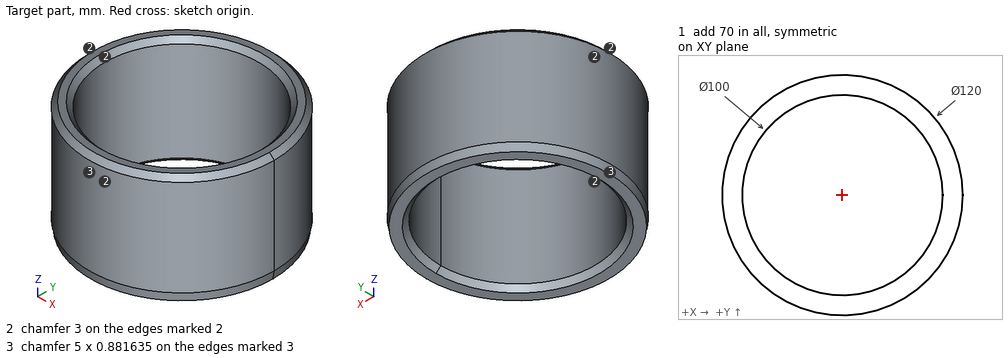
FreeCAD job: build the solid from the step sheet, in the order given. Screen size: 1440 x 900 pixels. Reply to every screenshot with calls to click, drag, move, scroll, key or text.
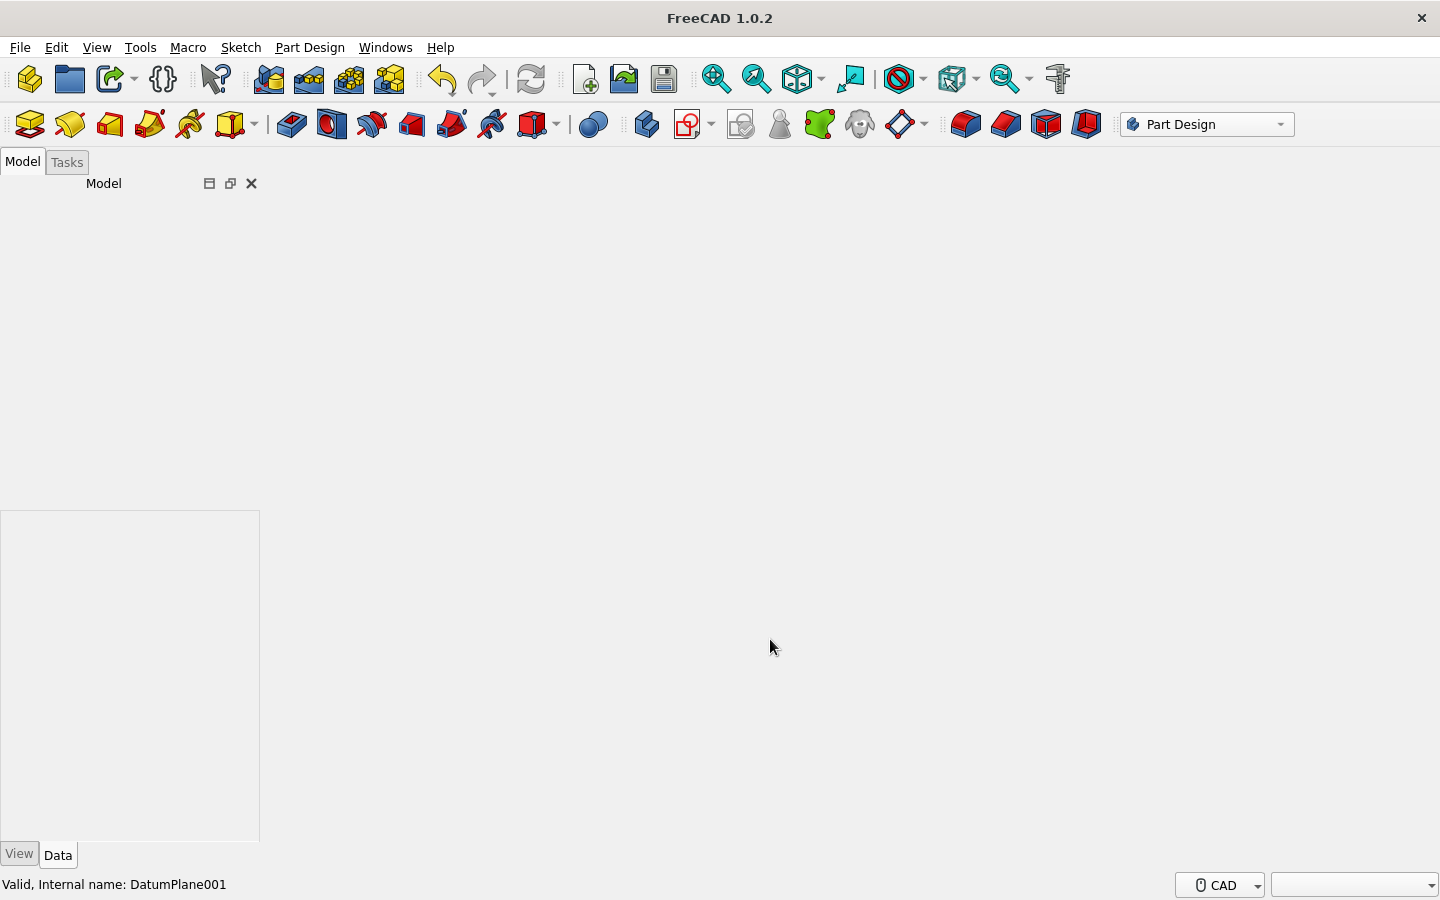
click(584, 80)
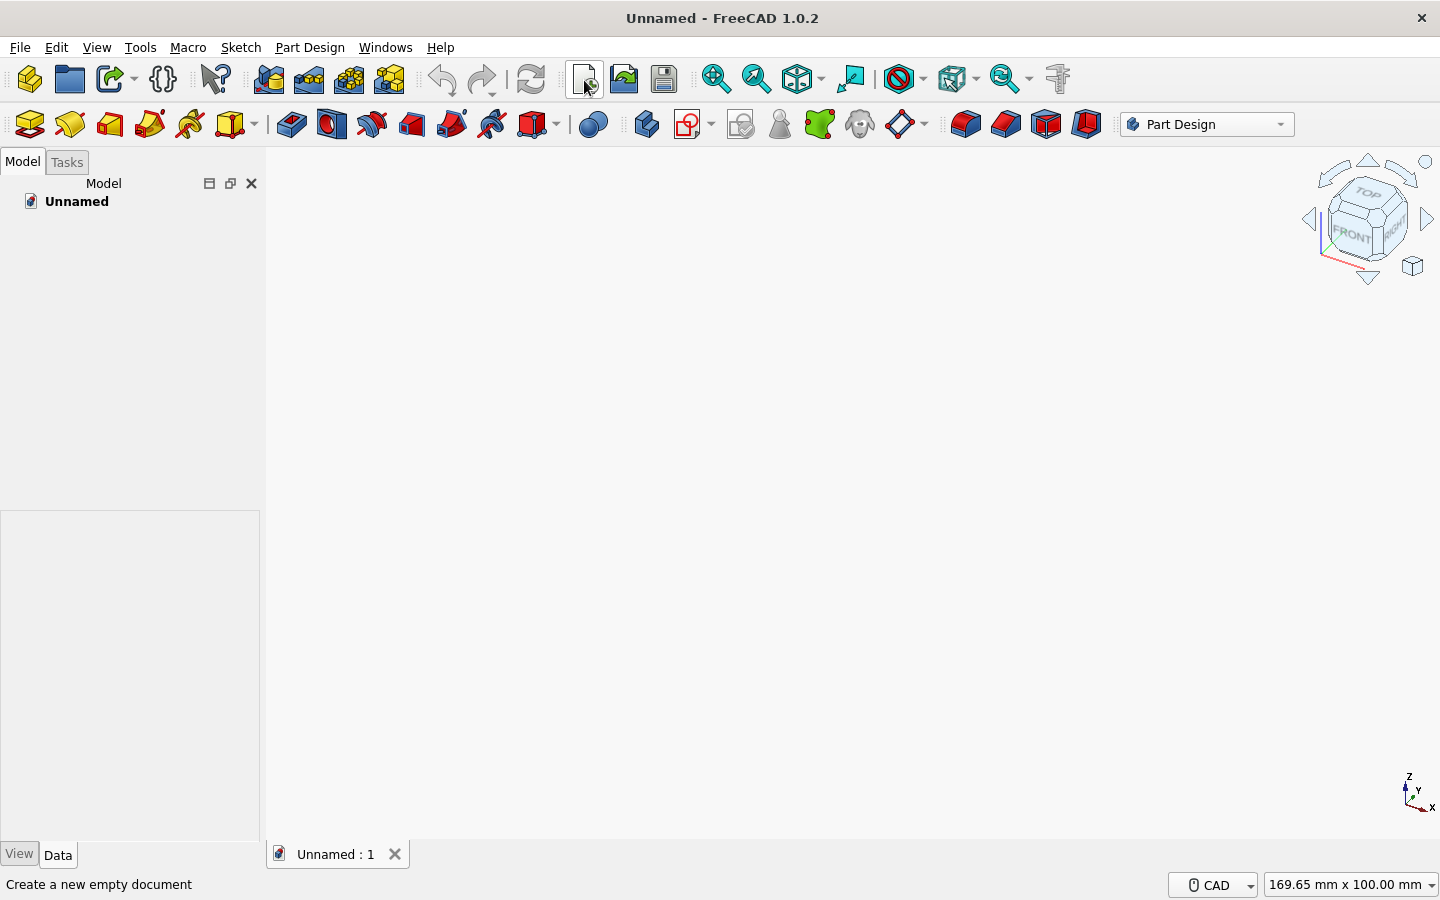
click(688, 124)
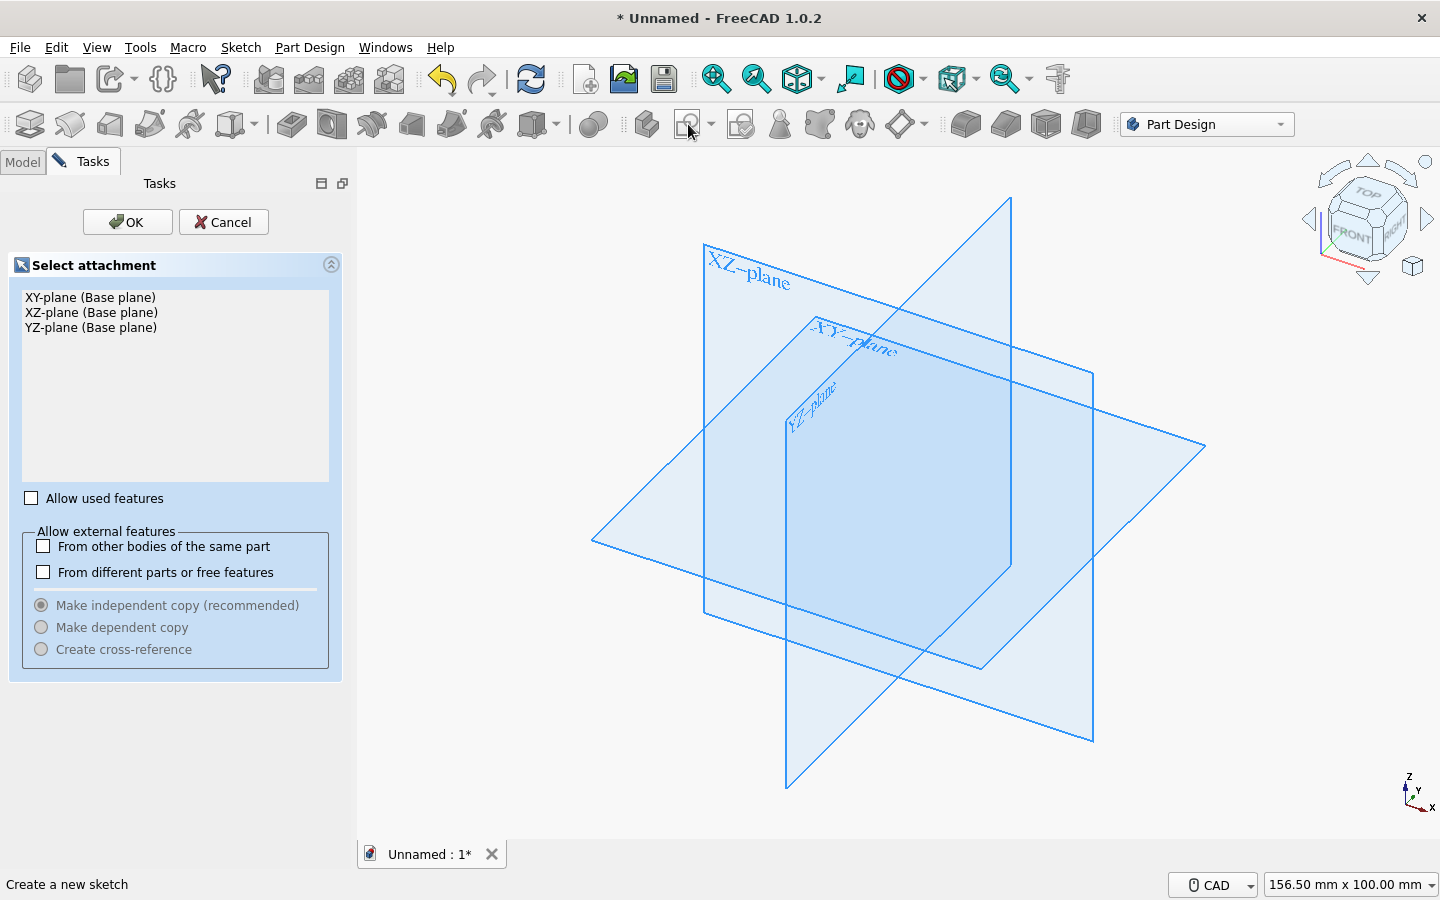
click(82, 298)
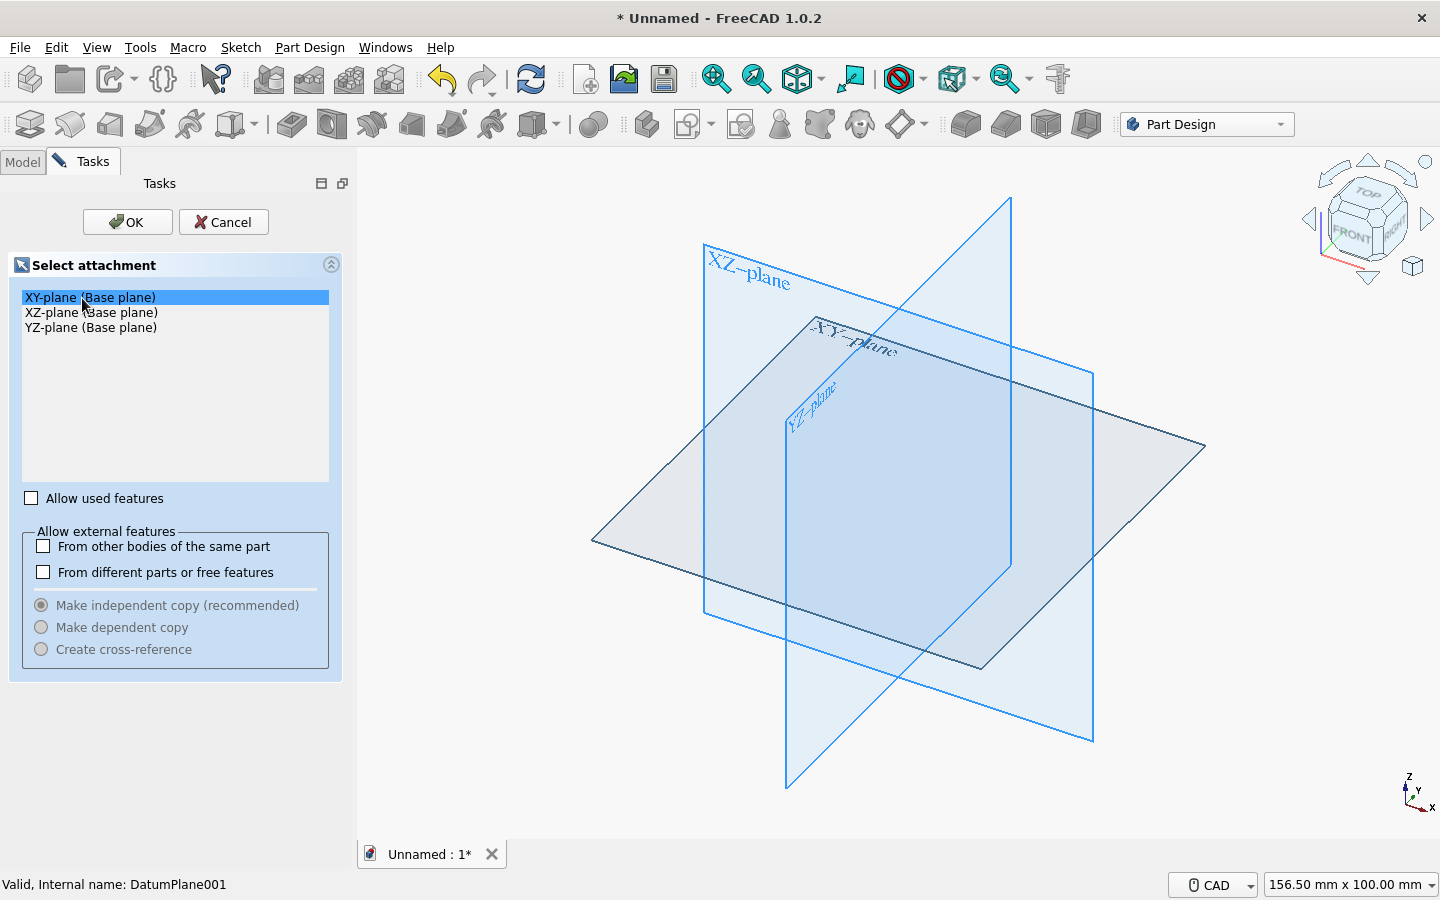
click(128, 222)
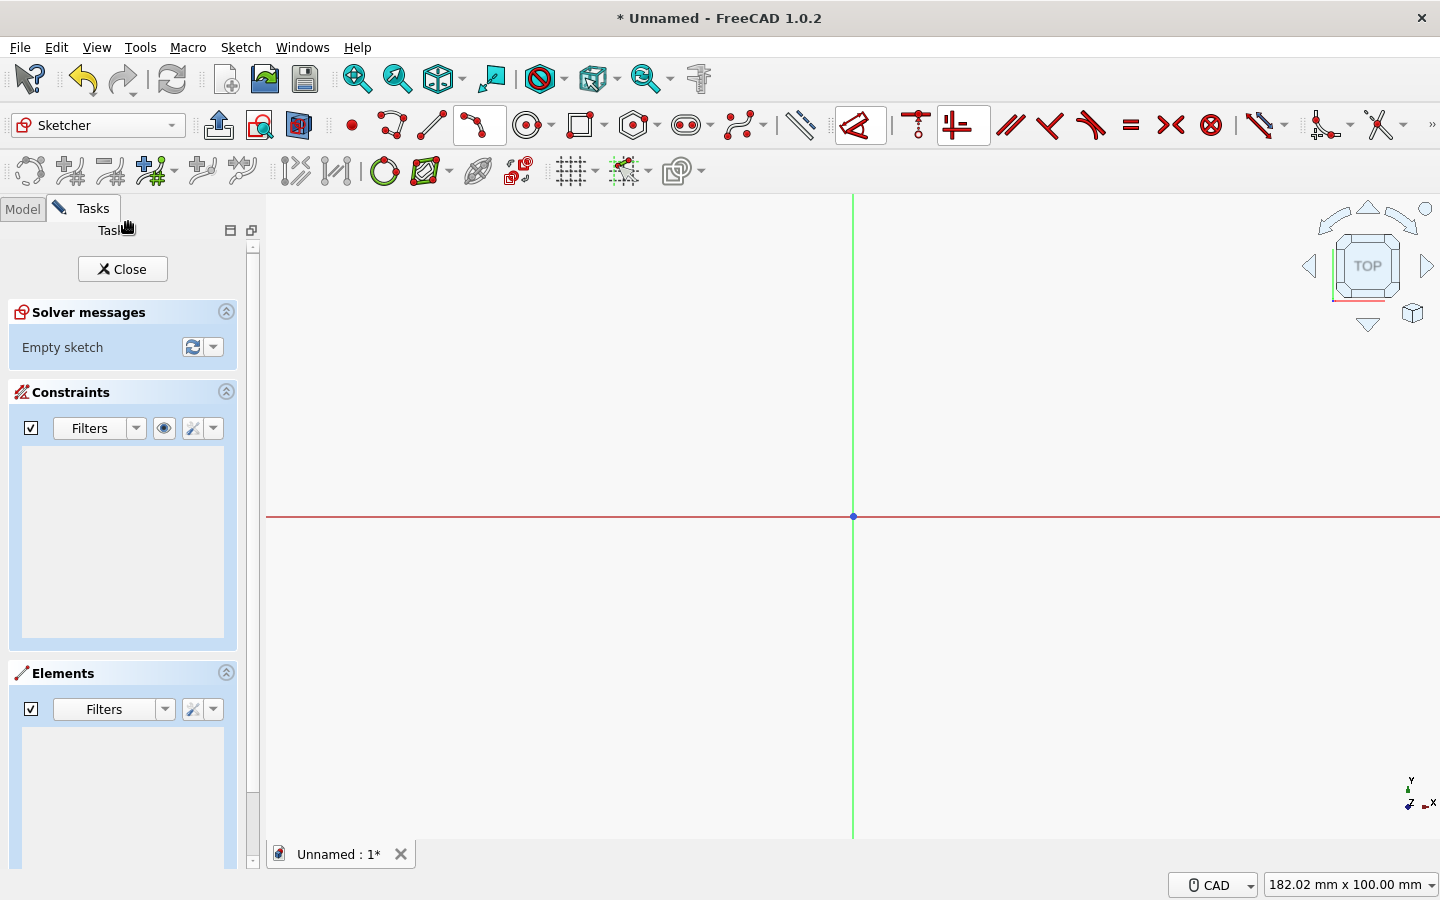
scroll(701, 516, down, 3)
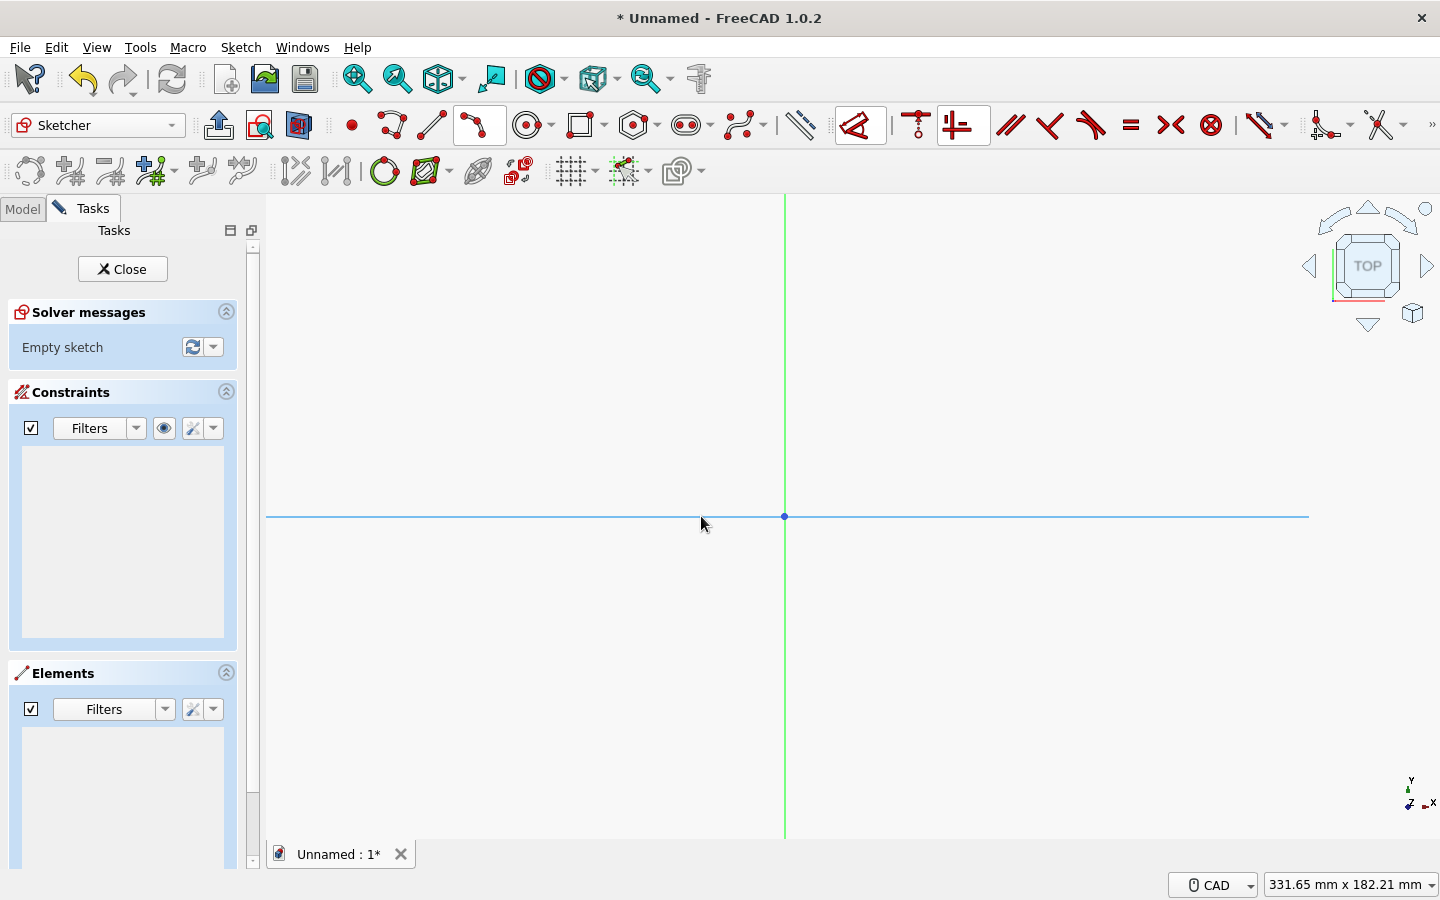
key(g)
key(c)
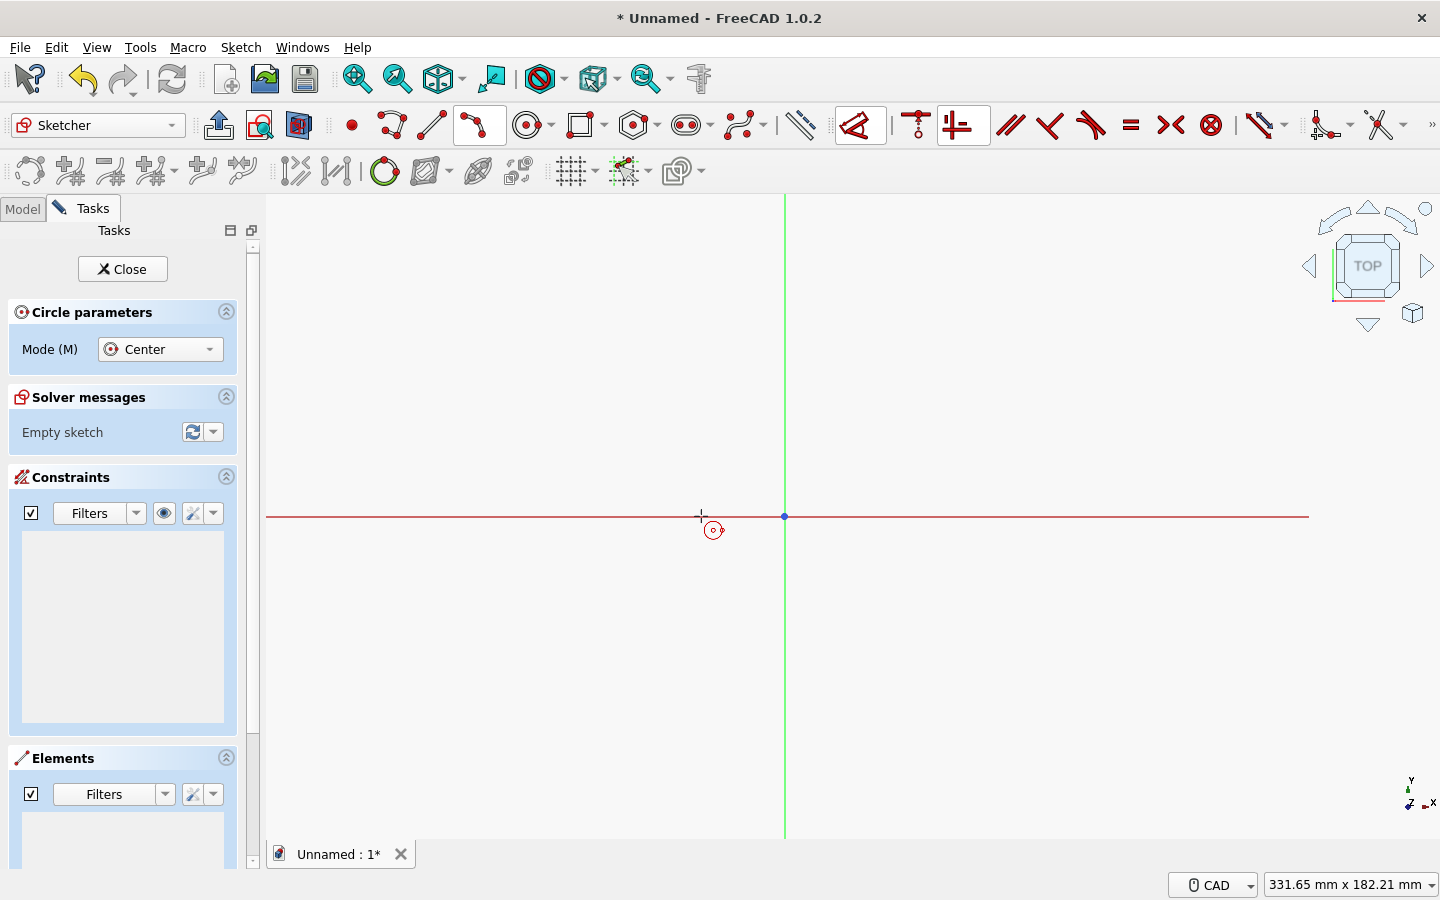
click(785, 516)
move(935, 366)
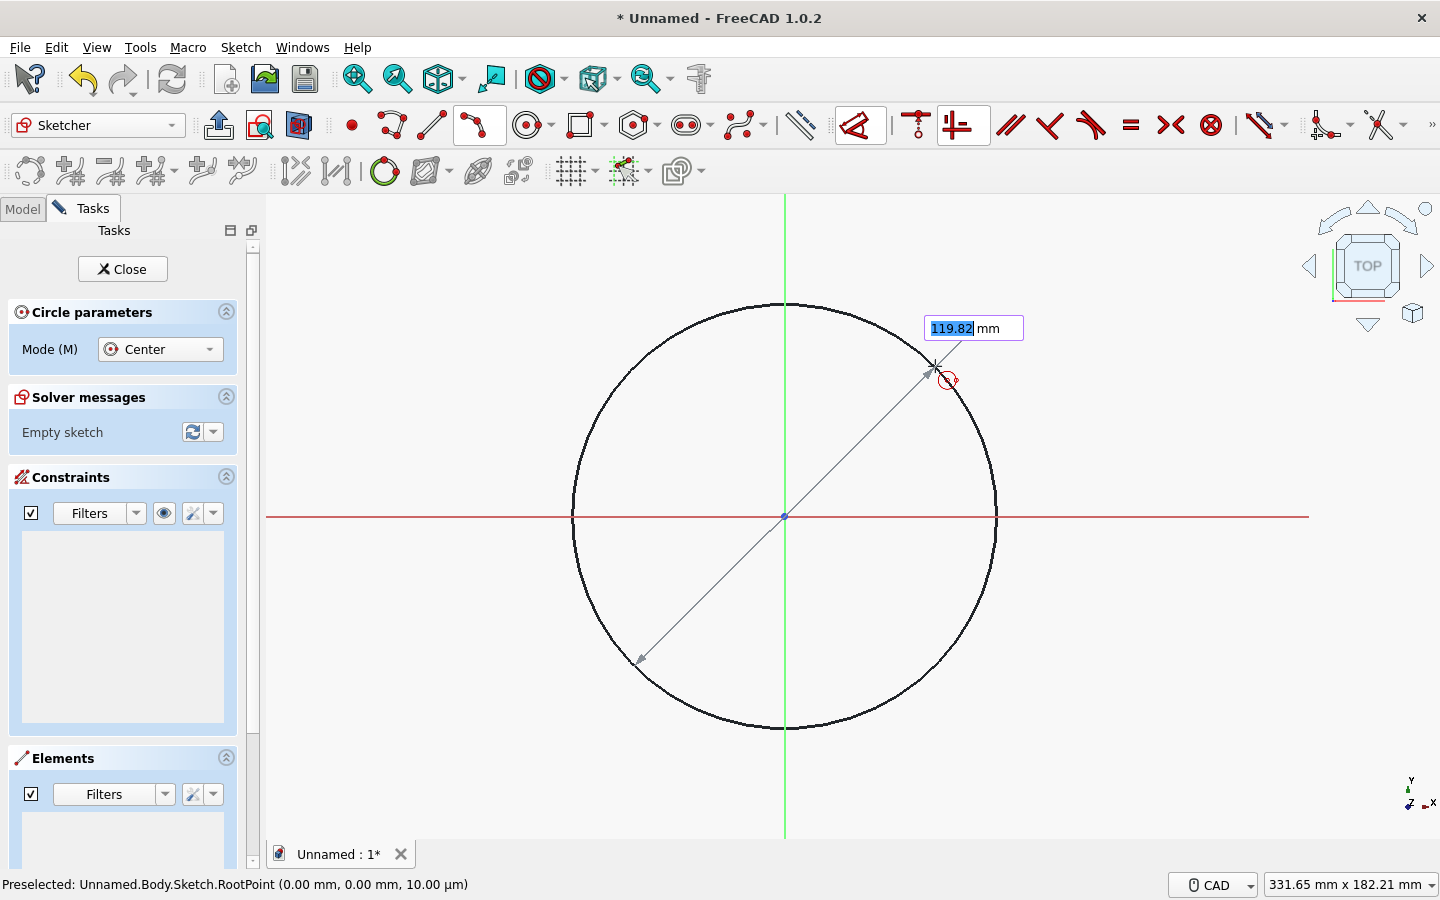
text(120)
key(Return)